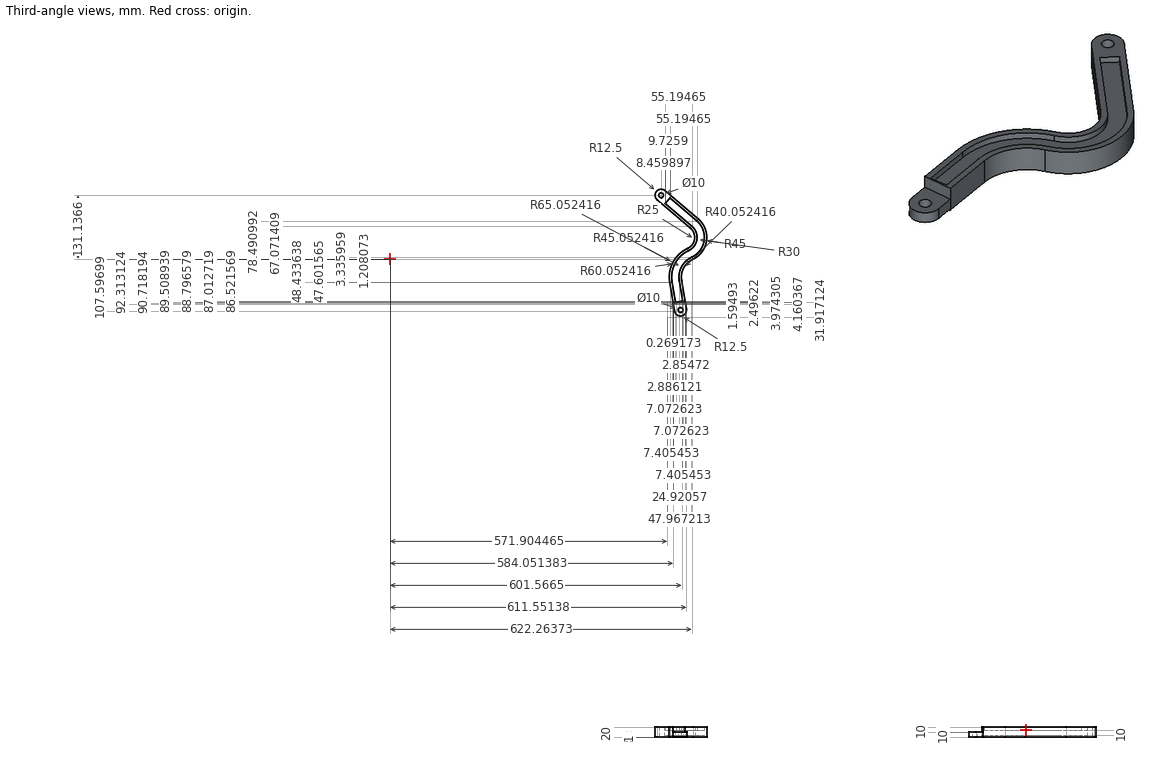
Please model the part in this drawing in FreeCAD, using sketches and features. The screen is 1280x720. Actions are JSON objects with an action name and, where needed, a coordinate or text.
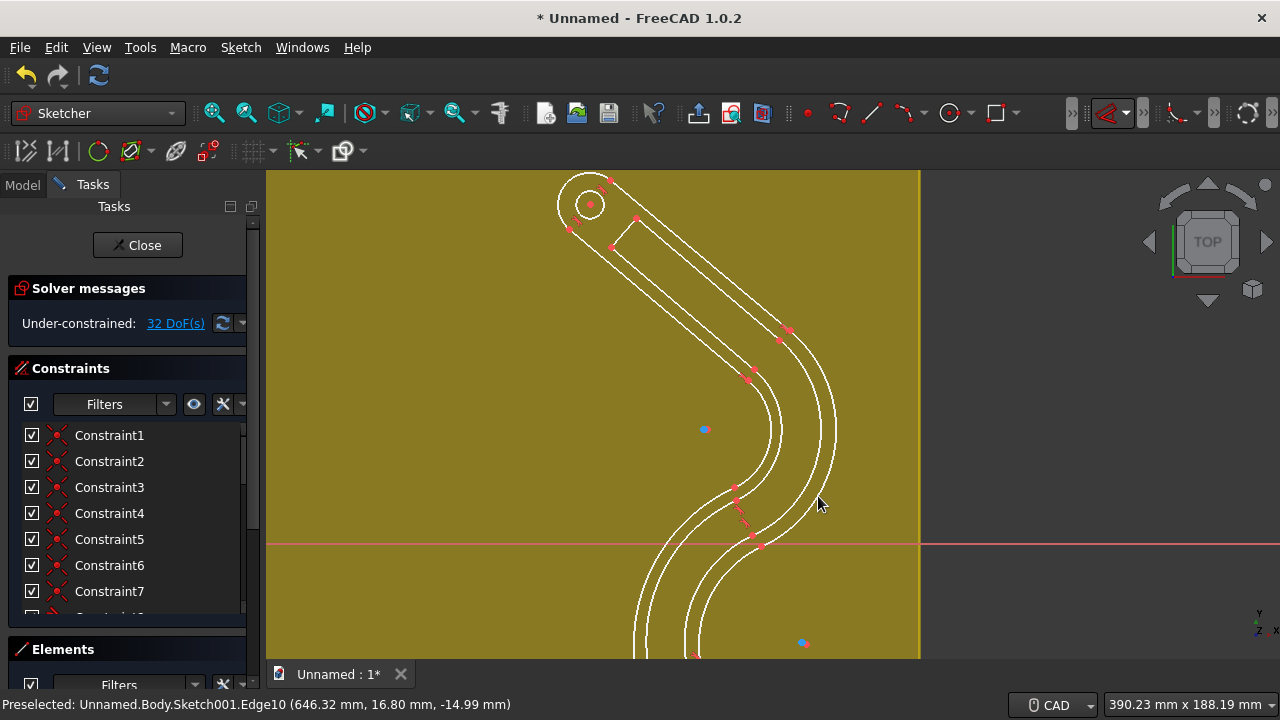
{"action": "left_click", "coordinate": [680, 527]}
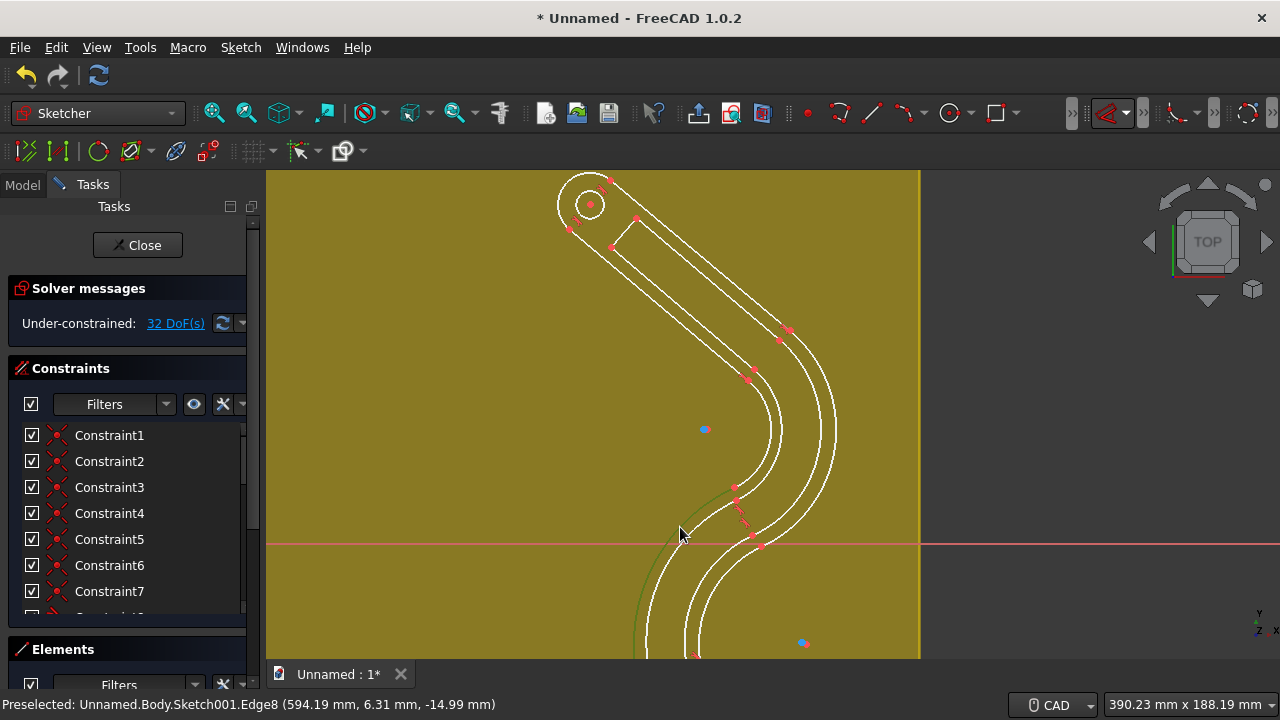
{"action": "left_click", "coordinate": [650, 607]}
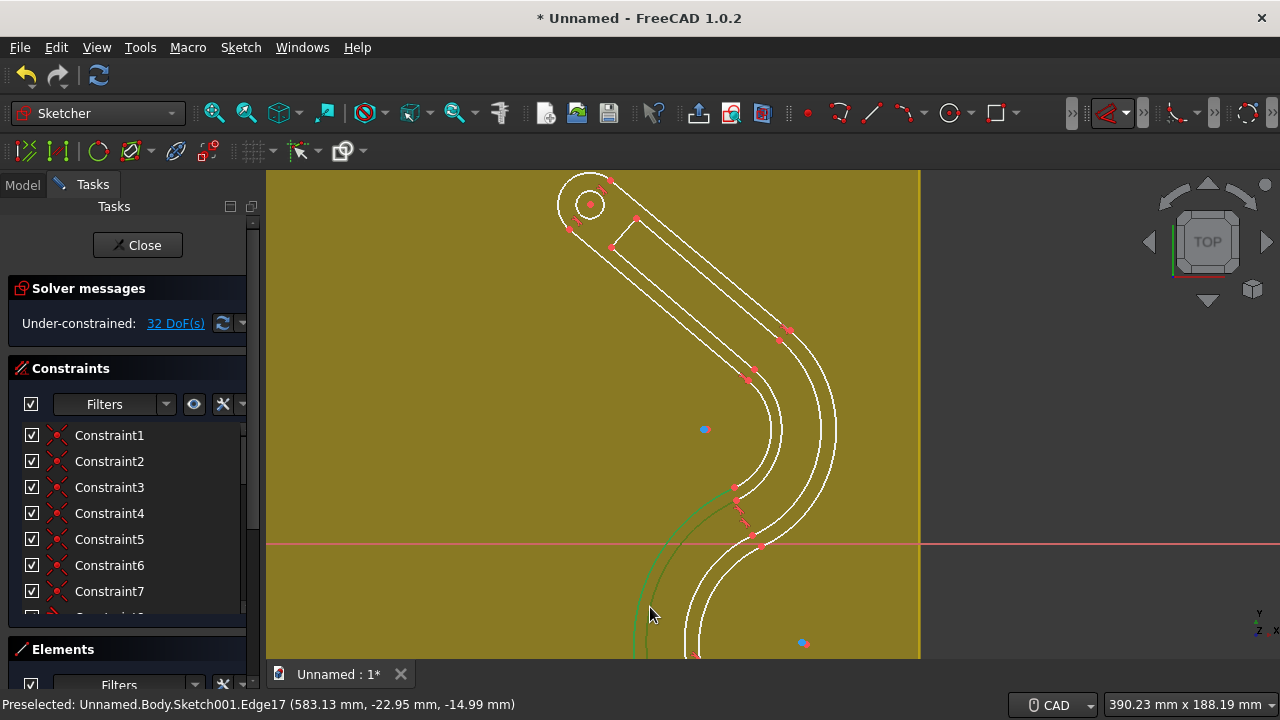
{"action": "key", "text": "c"}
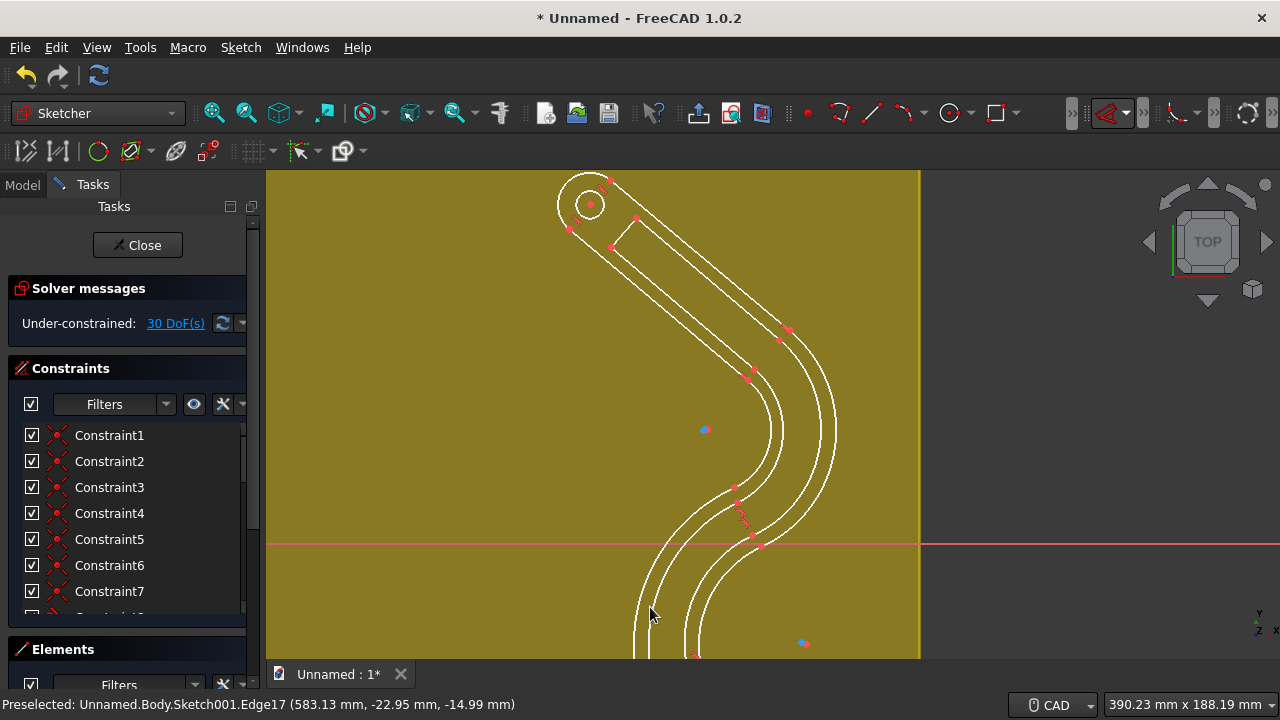
{"action": "left_click", "coordinate": [762, 463]}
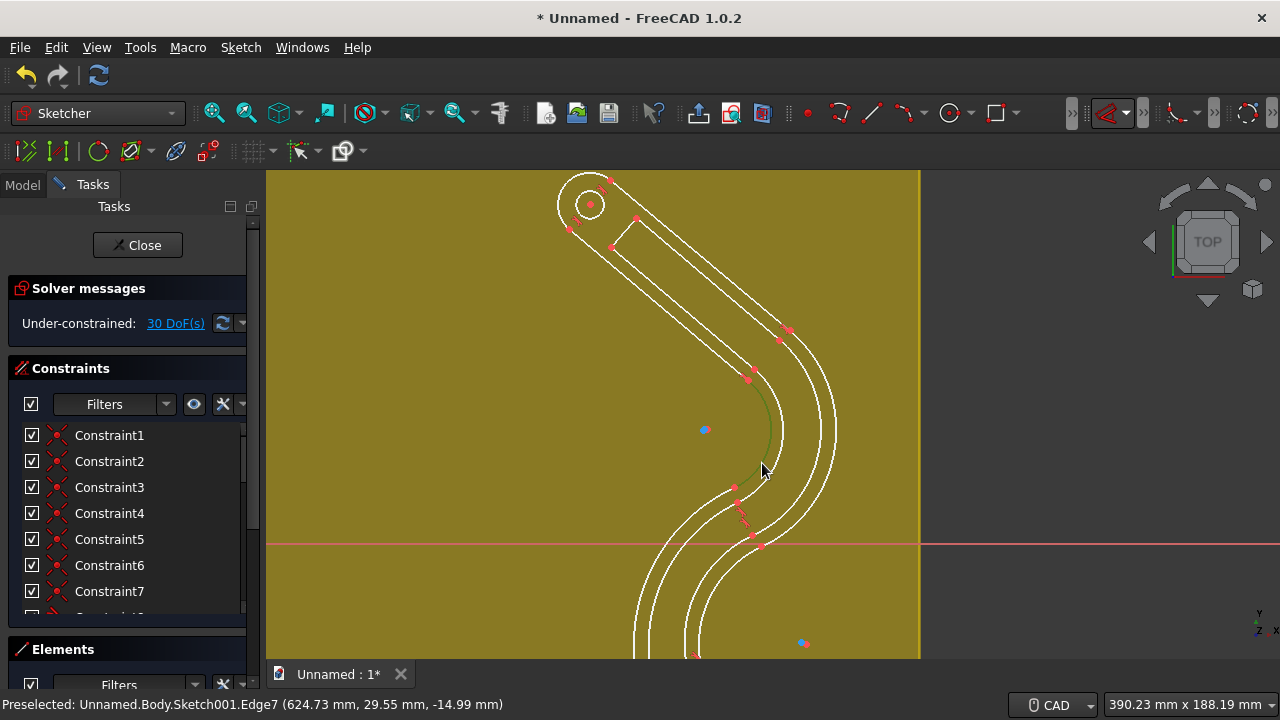
{"action": "left_click", "coordinate": [772, 471]}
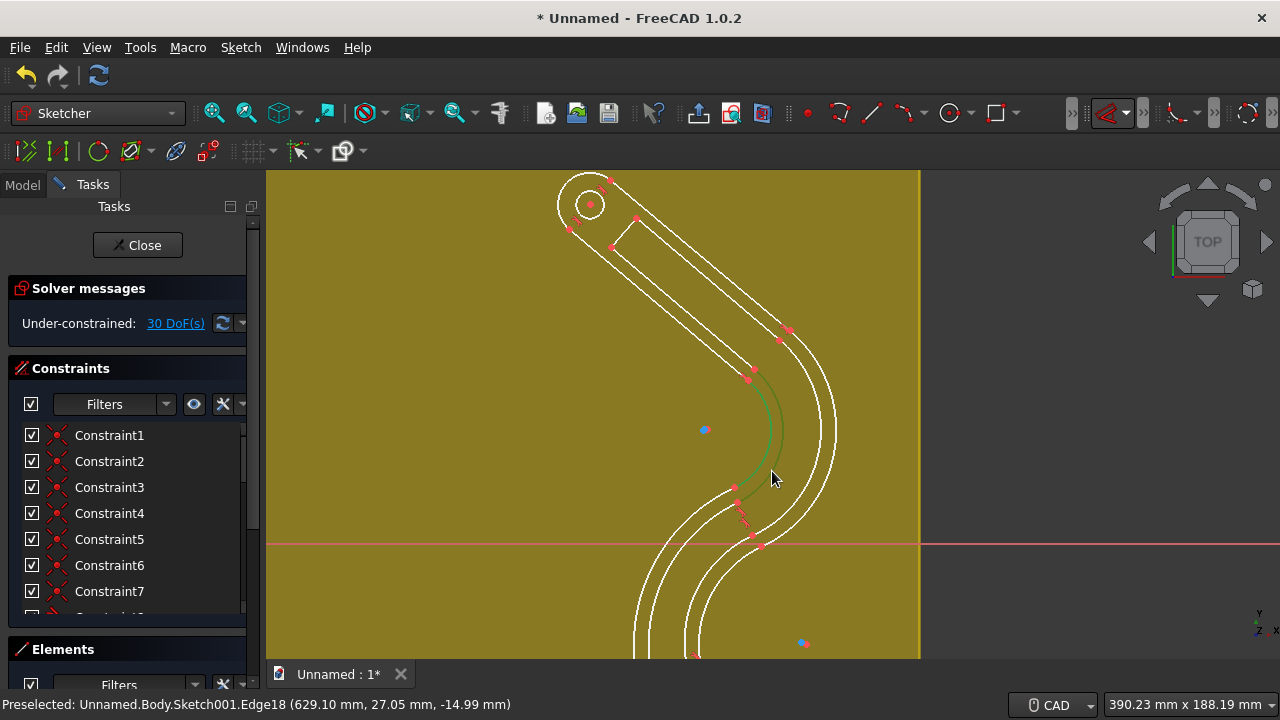
{"action": "key", "text": "c"}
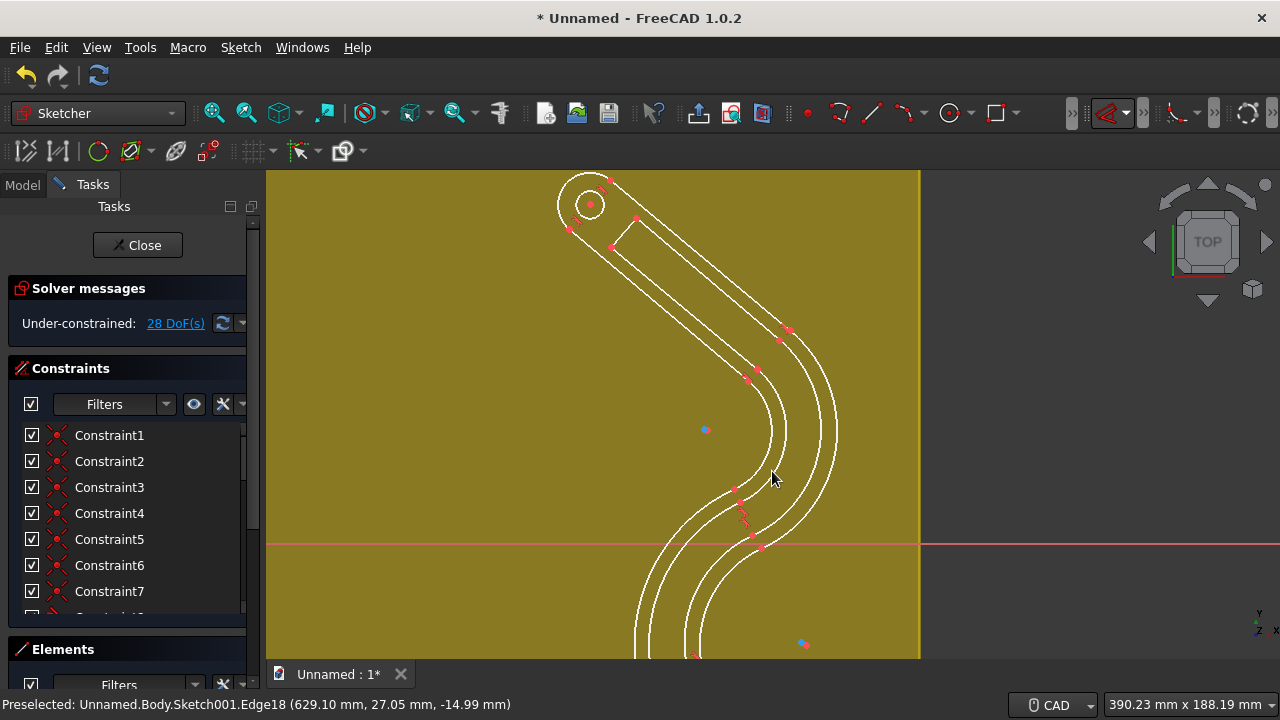
{"action": "left_click", "coordinate": [763, 464]}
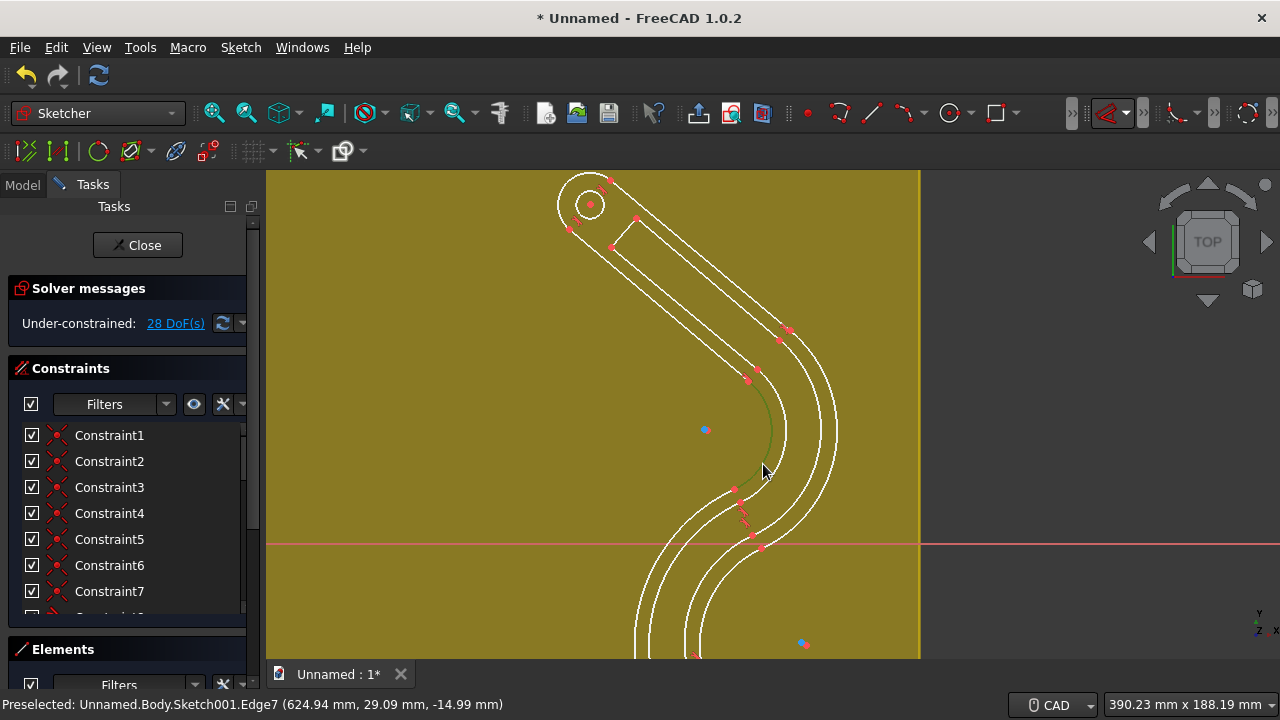
{"action": "left_click", "coordinate": [804, 489]}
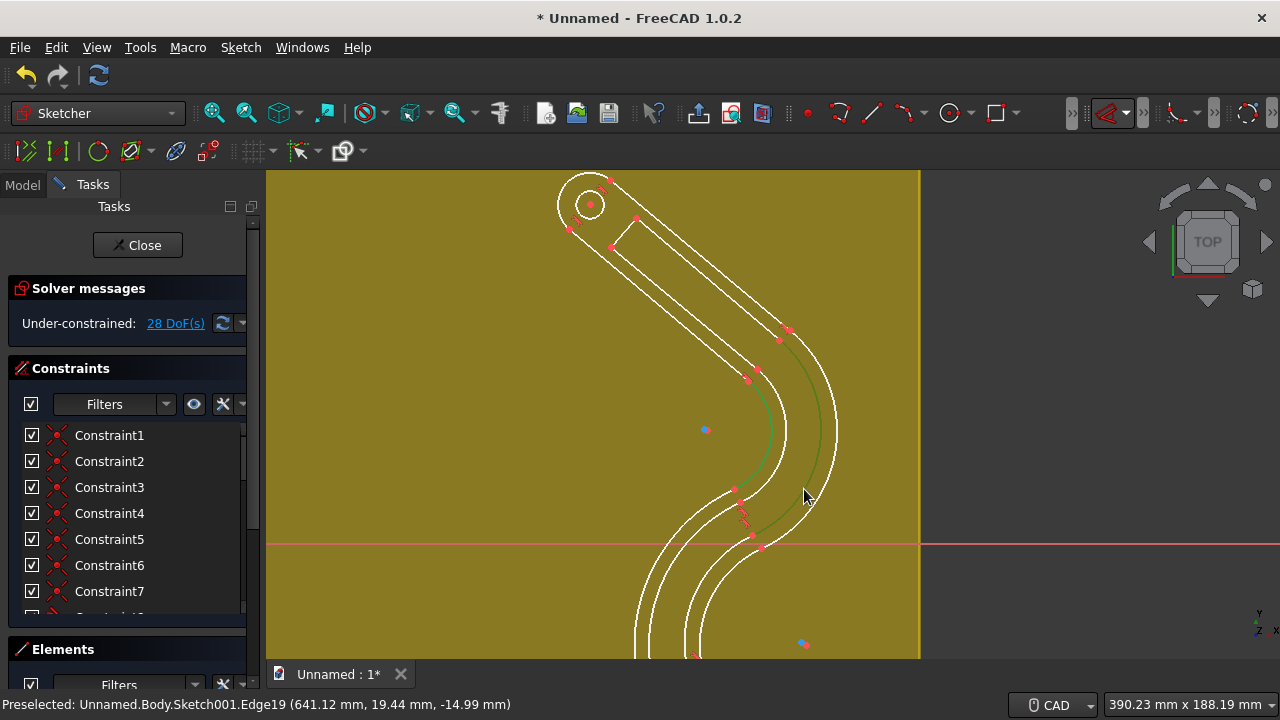
{"action": "key", "text": "c"}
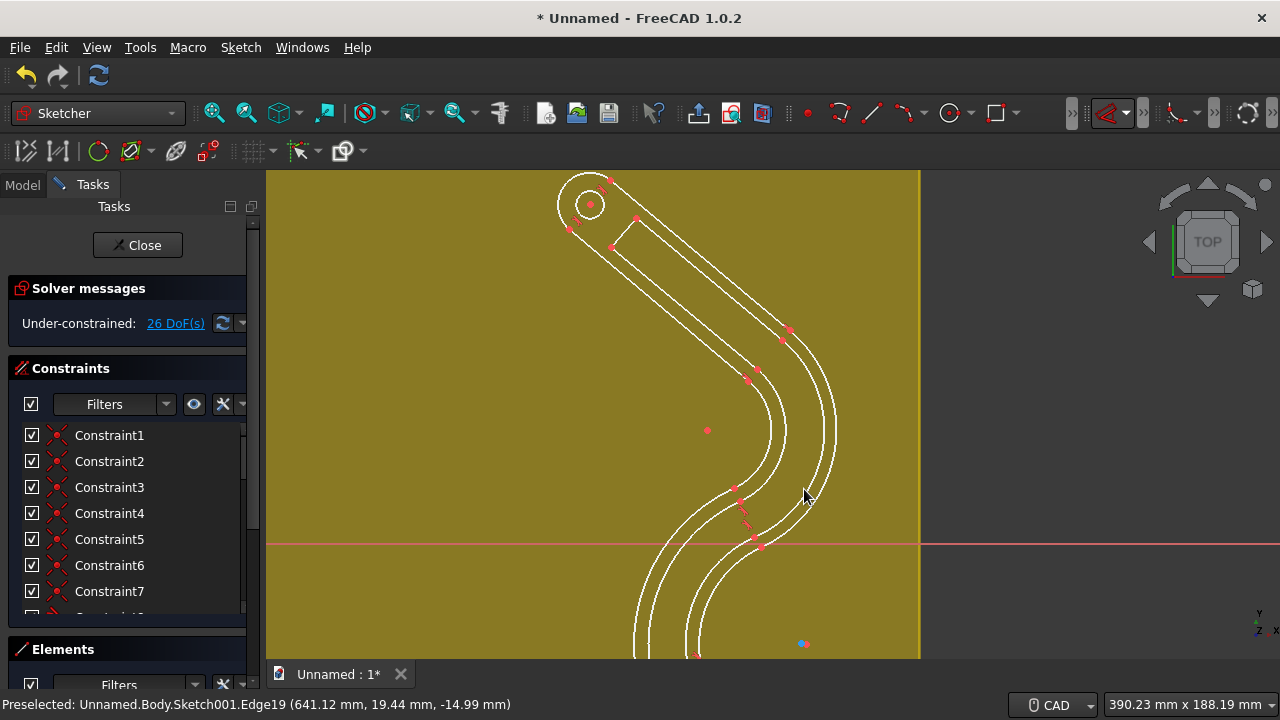
{"action": "left_click", "coordinate": [680, 527]}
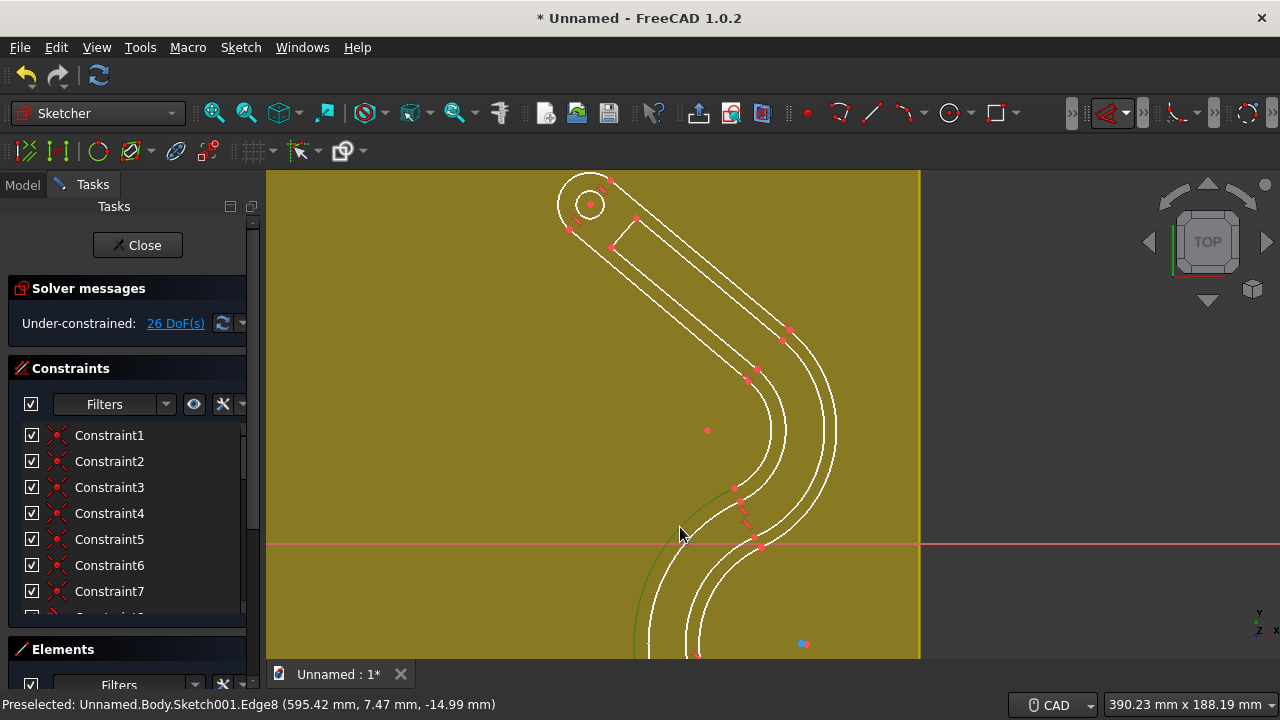
{"action": "left_click", "coordinate": [718, 563]}